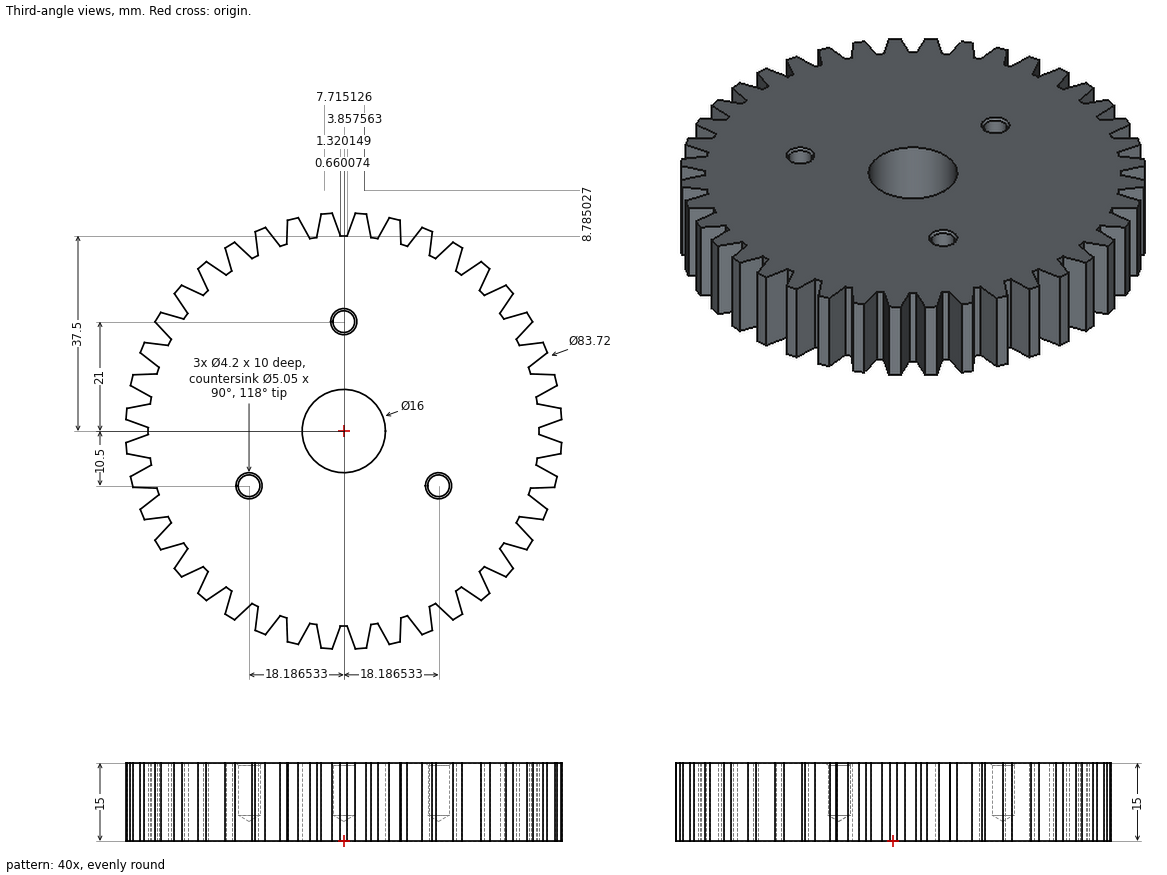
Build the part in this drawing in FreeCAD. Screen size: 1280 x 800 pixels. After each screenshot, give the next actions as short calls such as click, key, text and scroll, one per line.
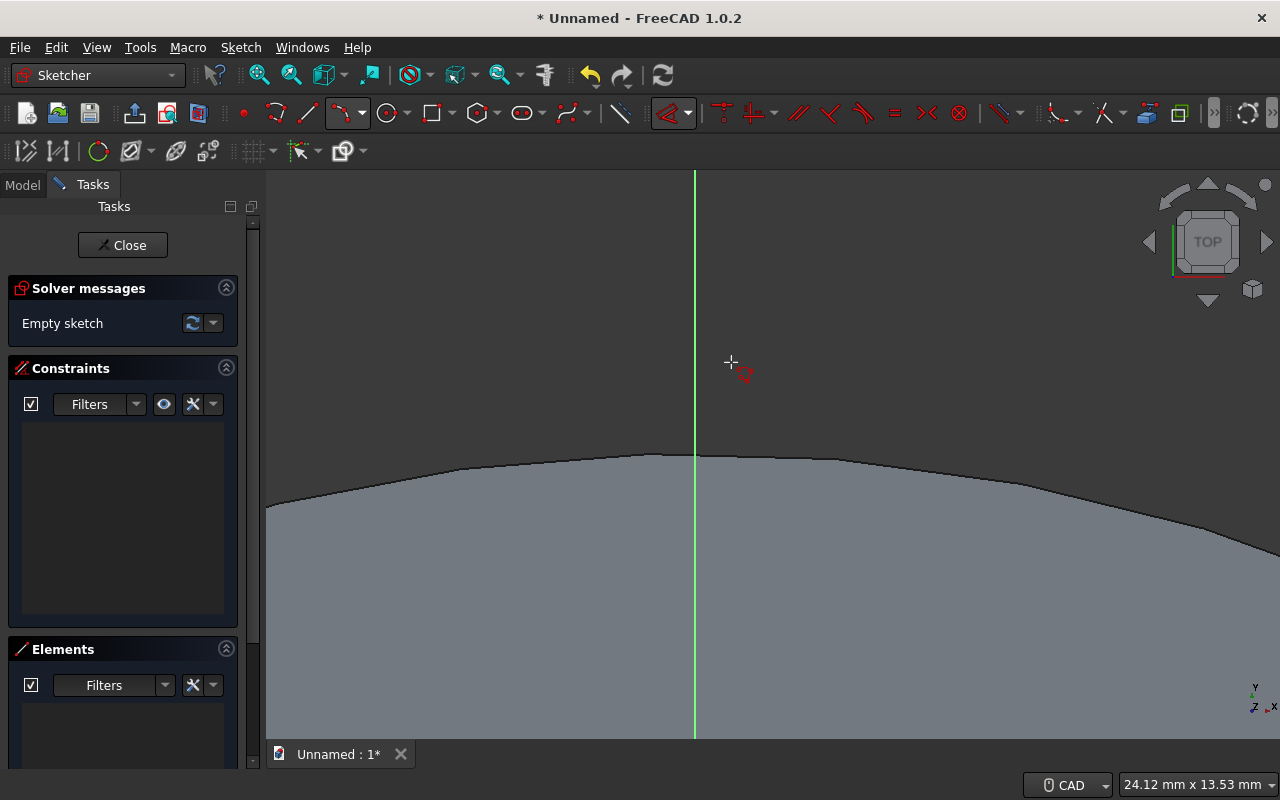
click(668, 637)
click(723, 637)
click(857, 267)
click(533, 267)
click(668, 638)
key(Escape)
key(Escape)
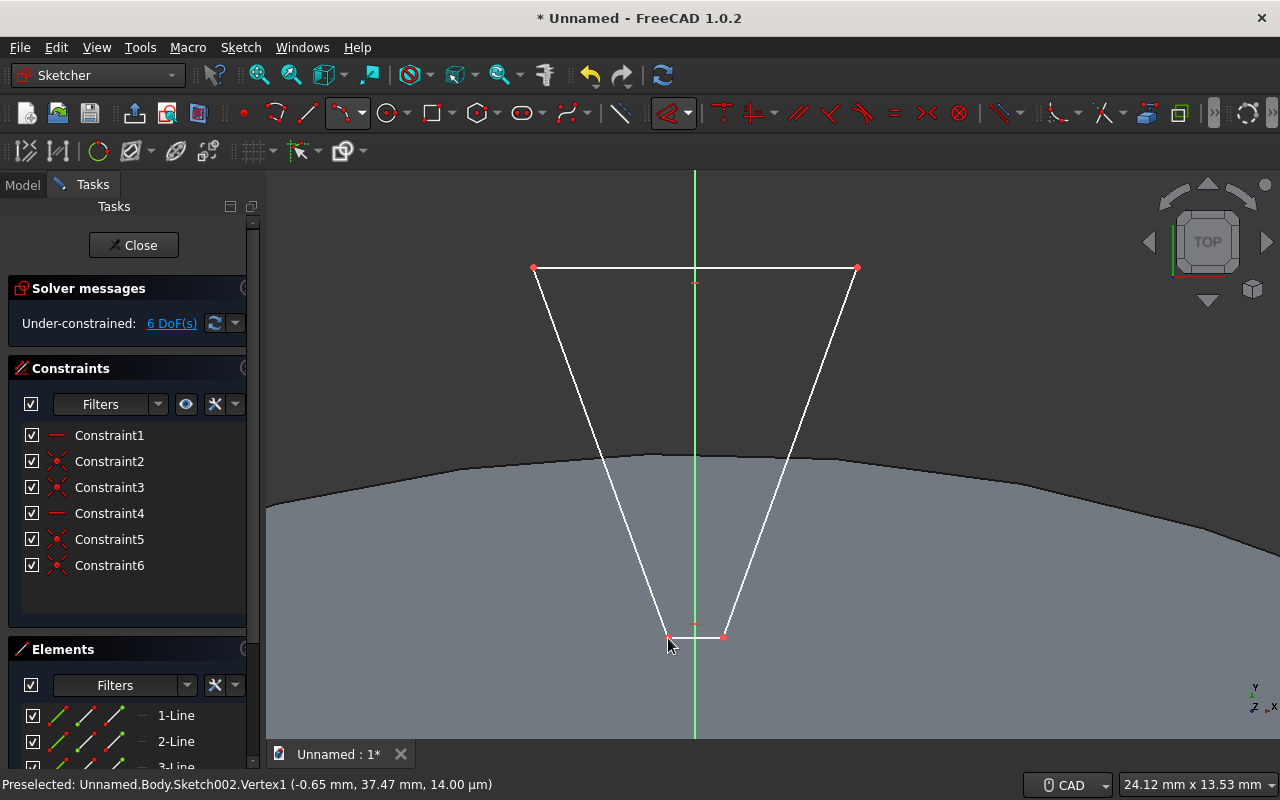
key(d)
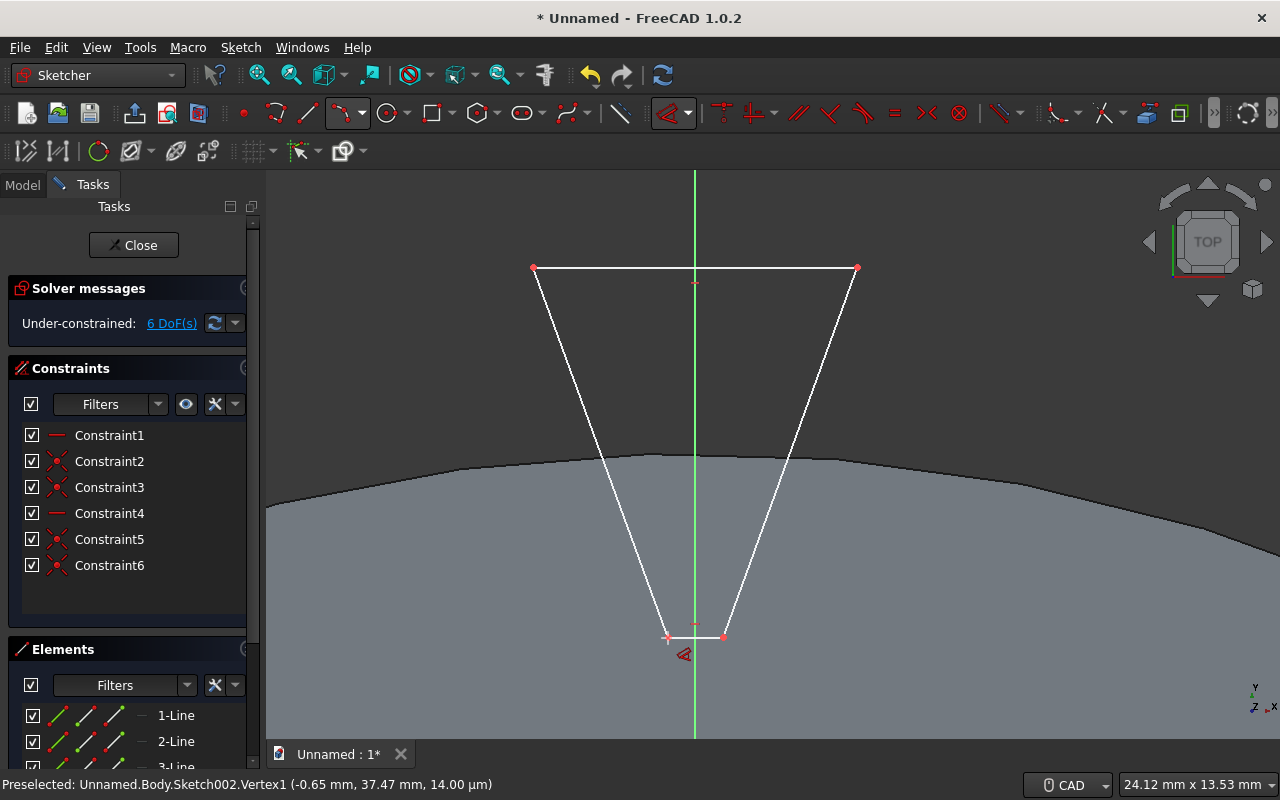
click(668, 638)
click(634, 675)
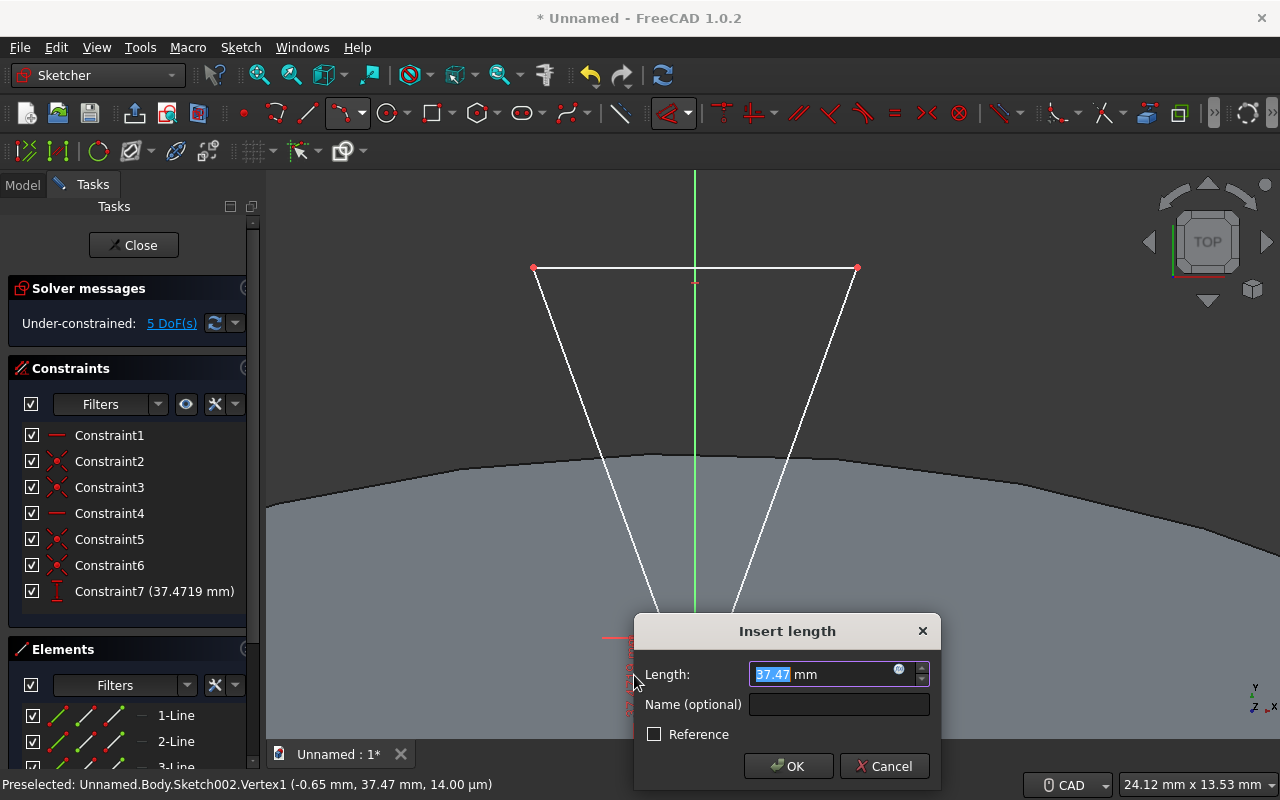
text(37.5)
key(Return)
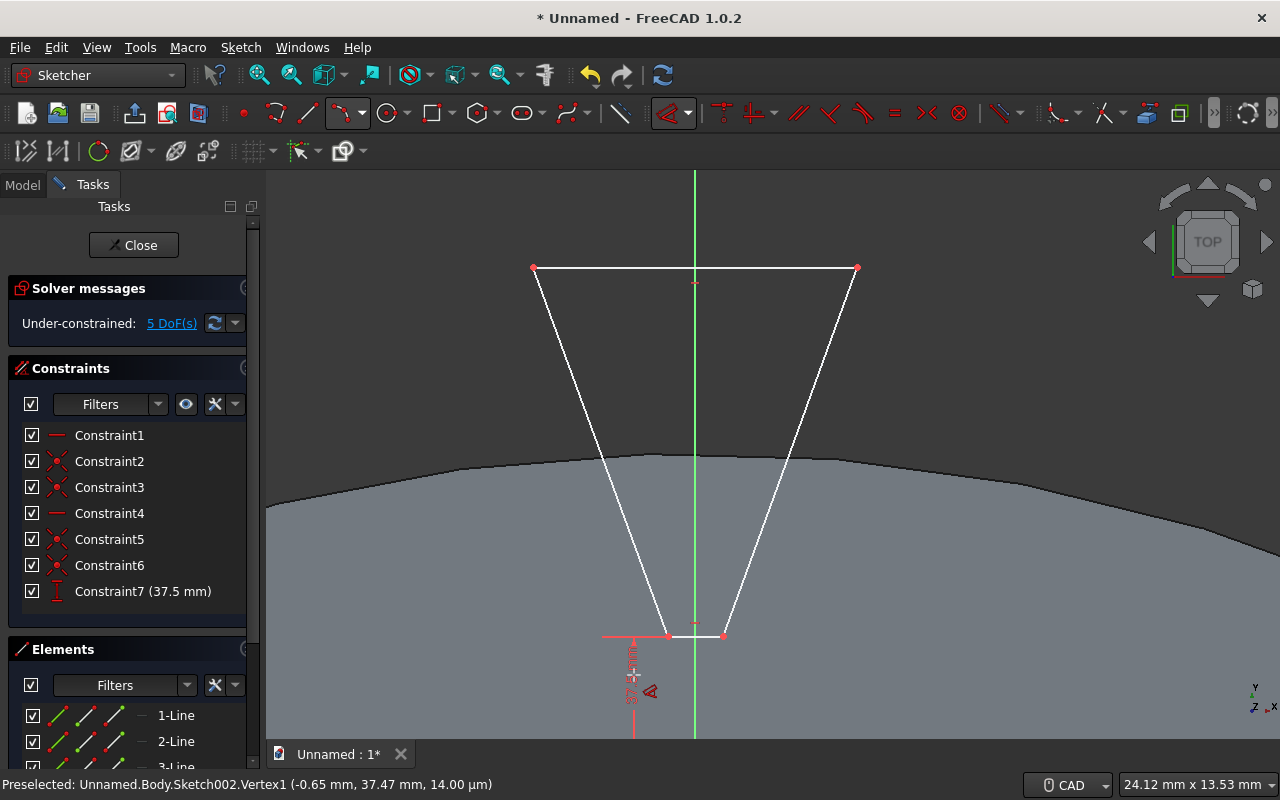
scroll(685, 637, up, 2)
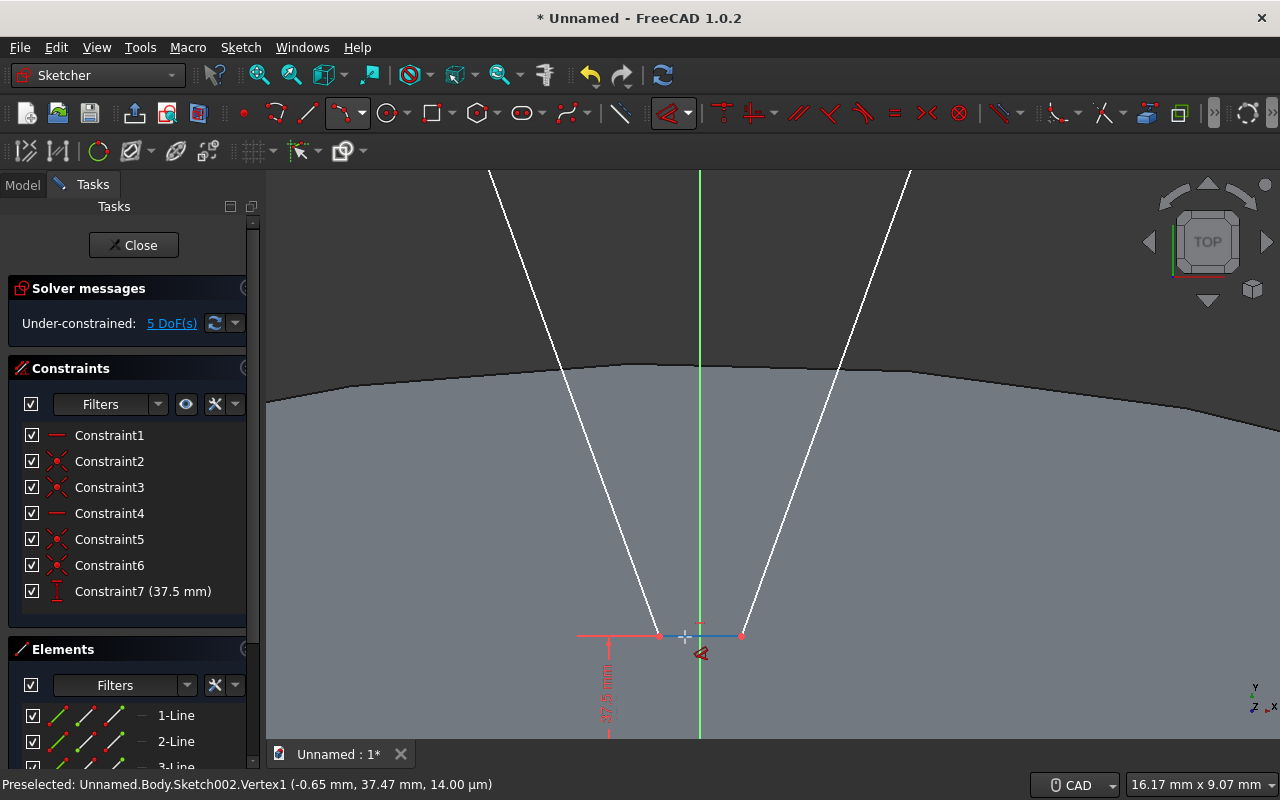
click(684, 636)
click(682, 670)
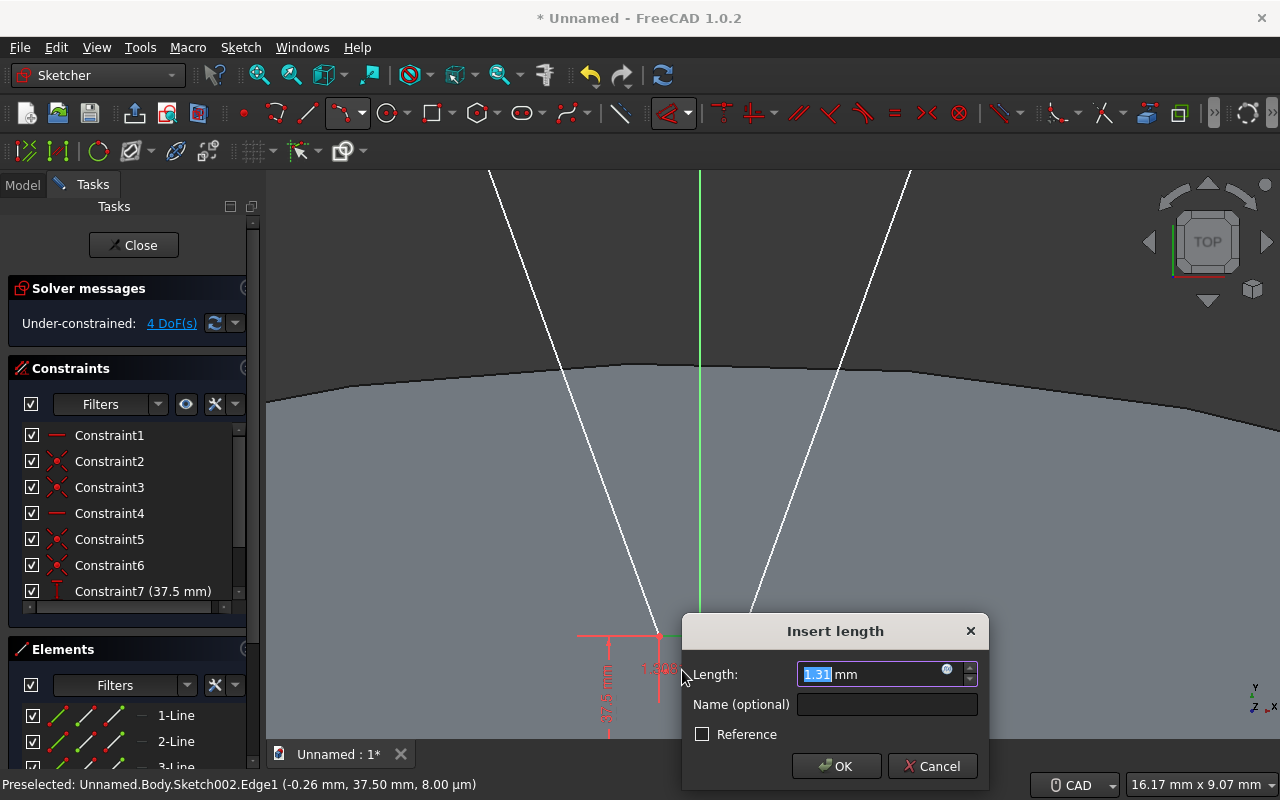
text(1.320149)
key(Return)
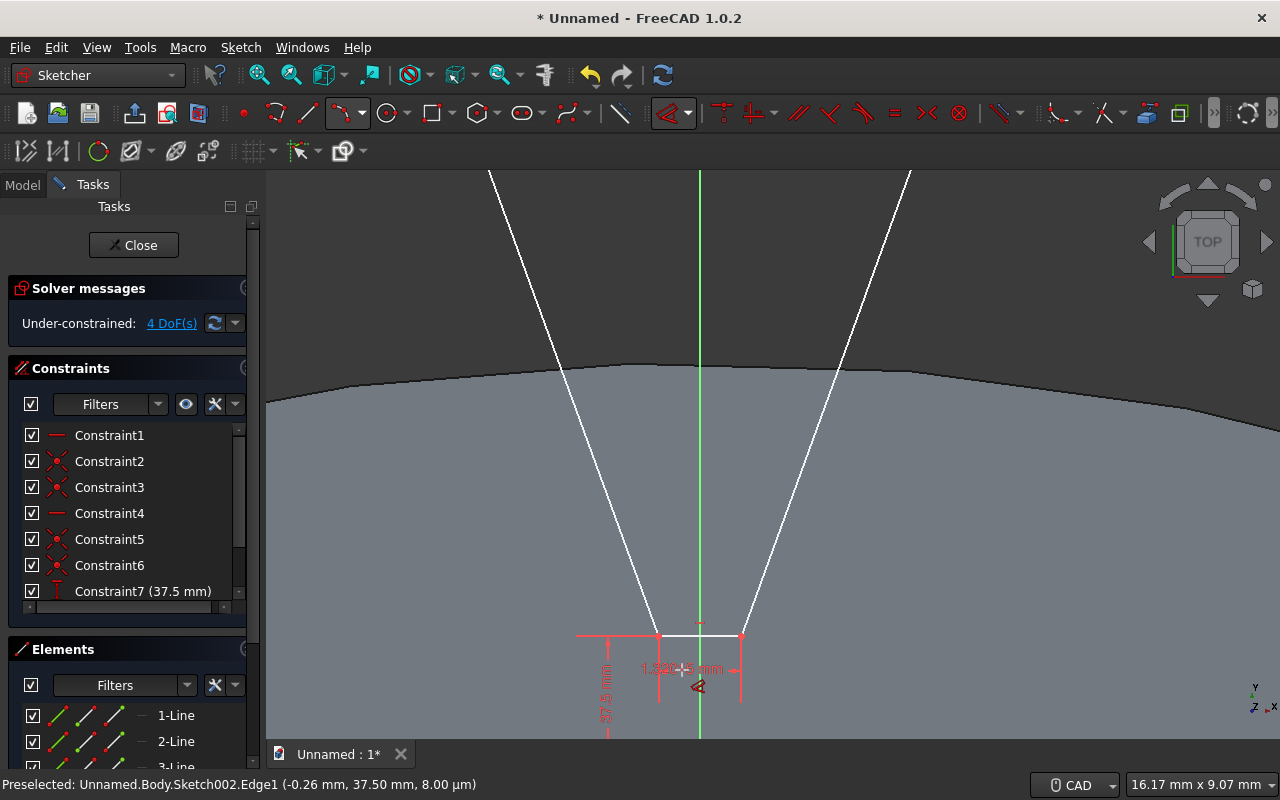
scroll(713, 645, down, 2)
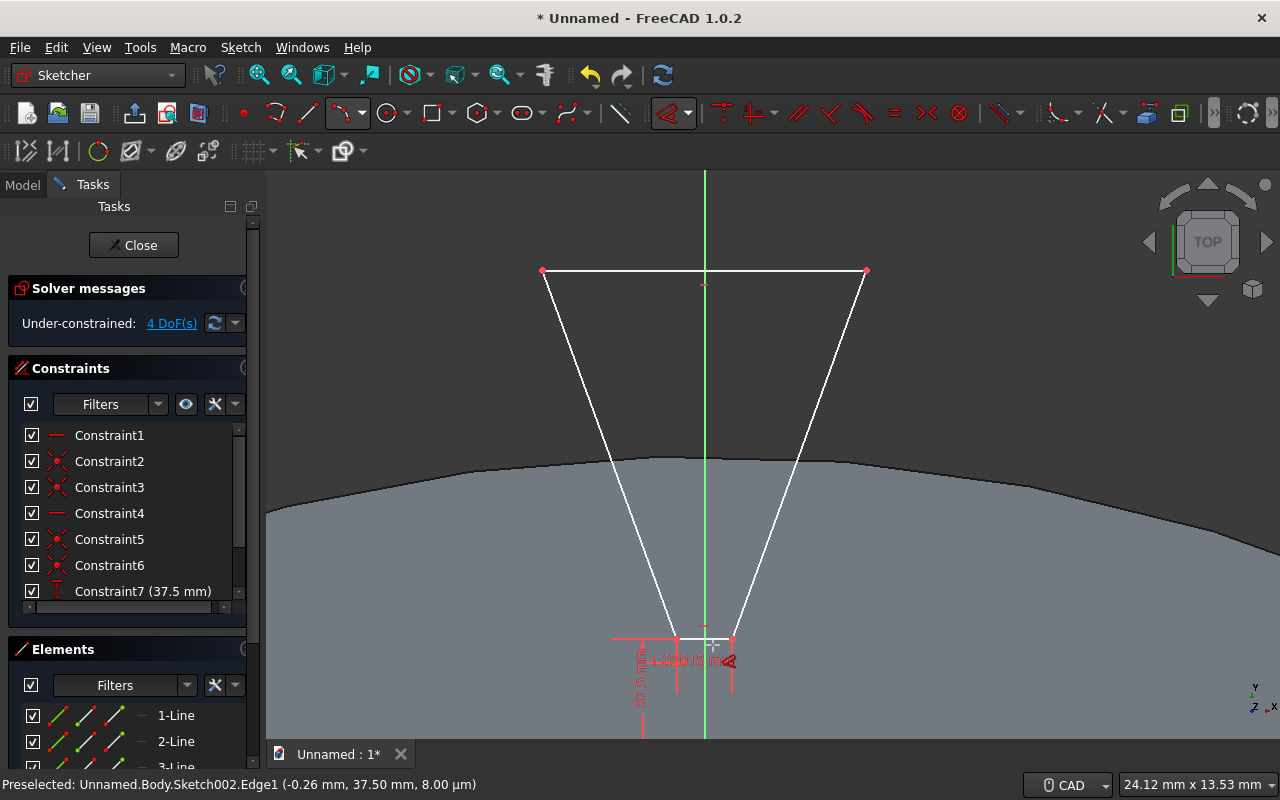
click(769, 271)
click(630, 237)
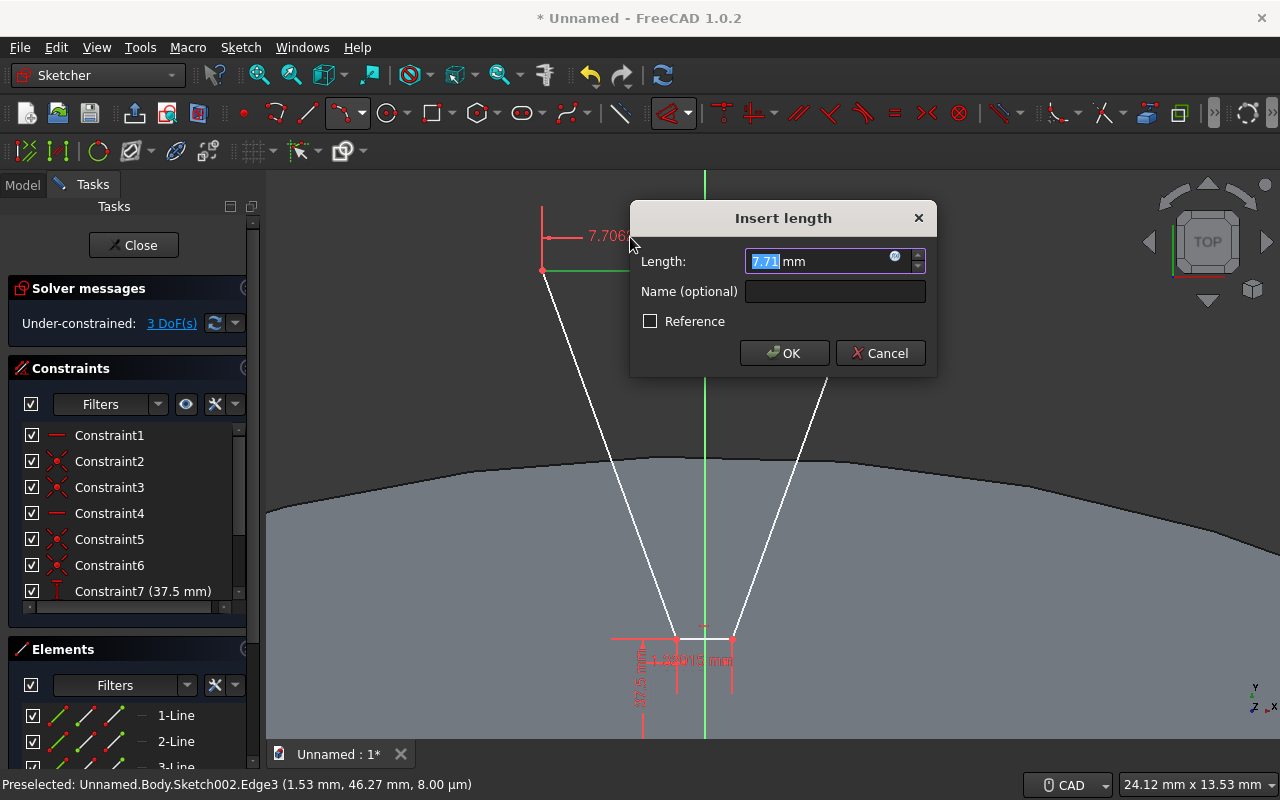
text(7.715126)
key(Return)